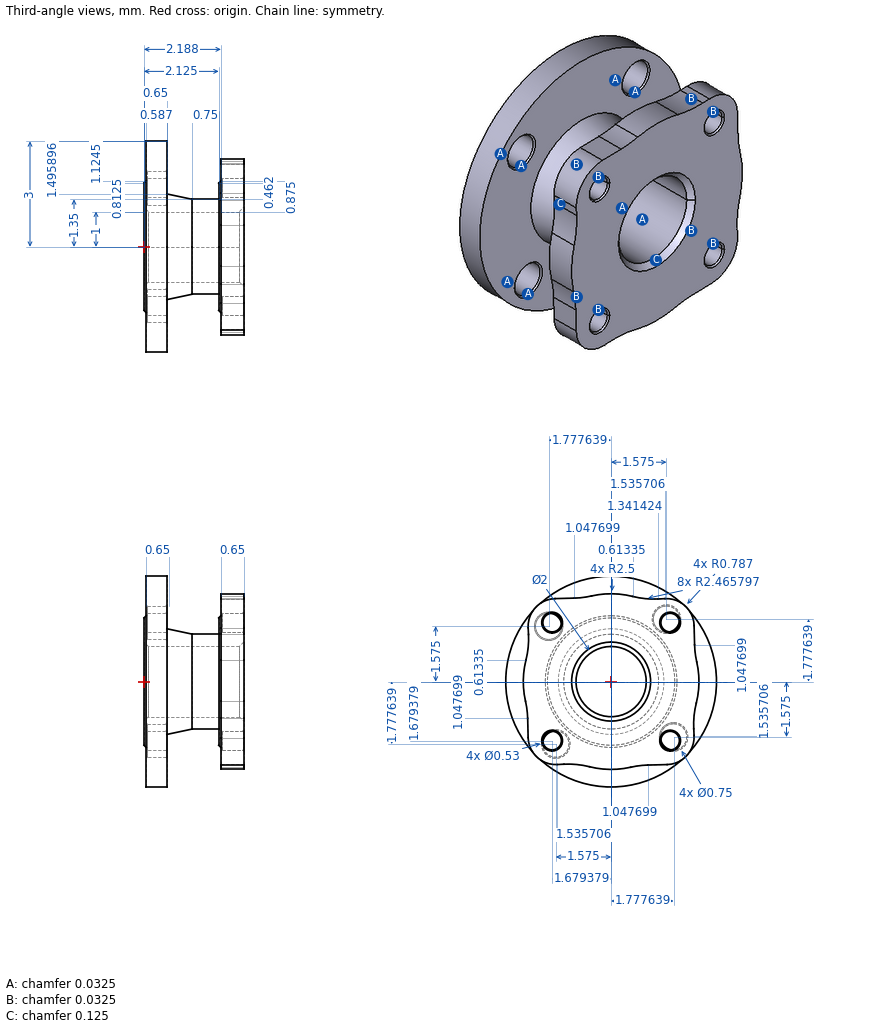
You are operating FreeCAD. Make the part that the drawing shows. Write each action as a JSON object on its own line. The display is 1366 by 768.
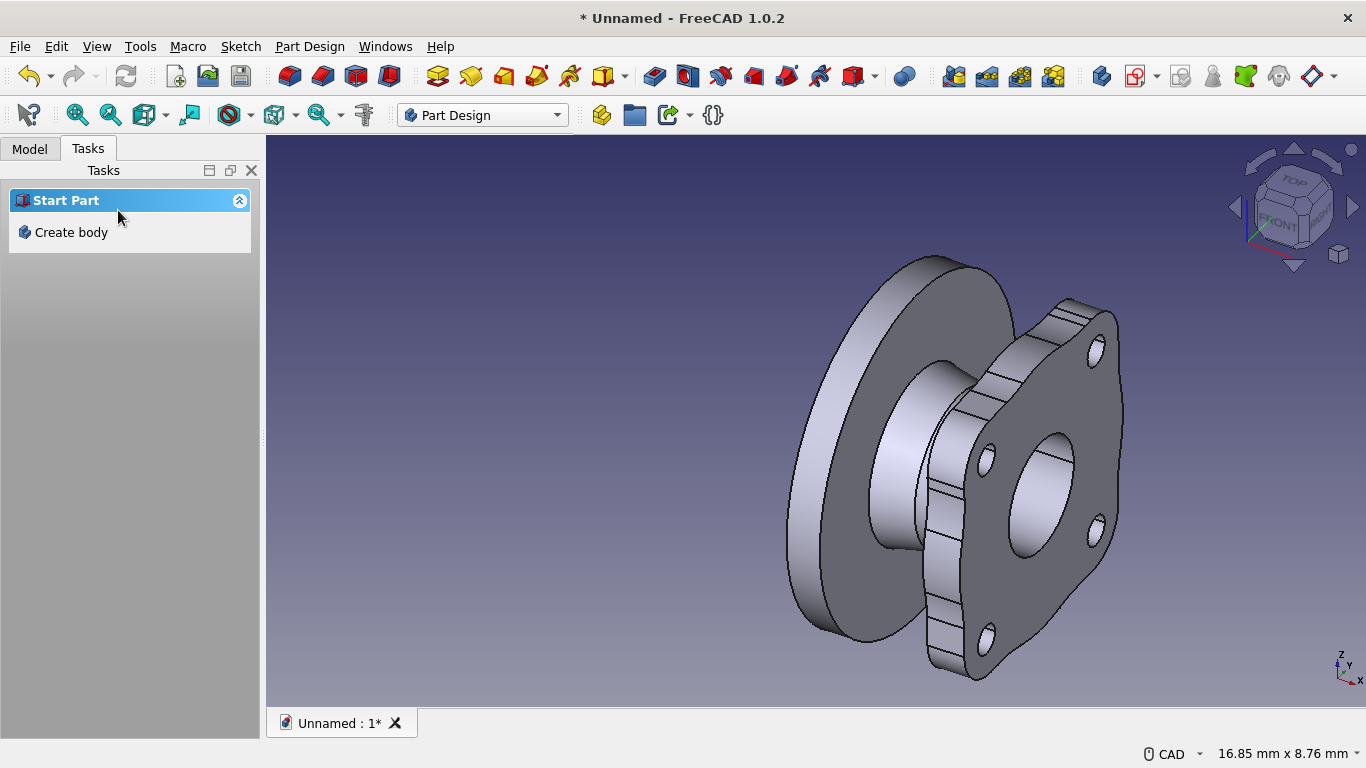
{"action": "left_click", "coordinate": [78, 116]}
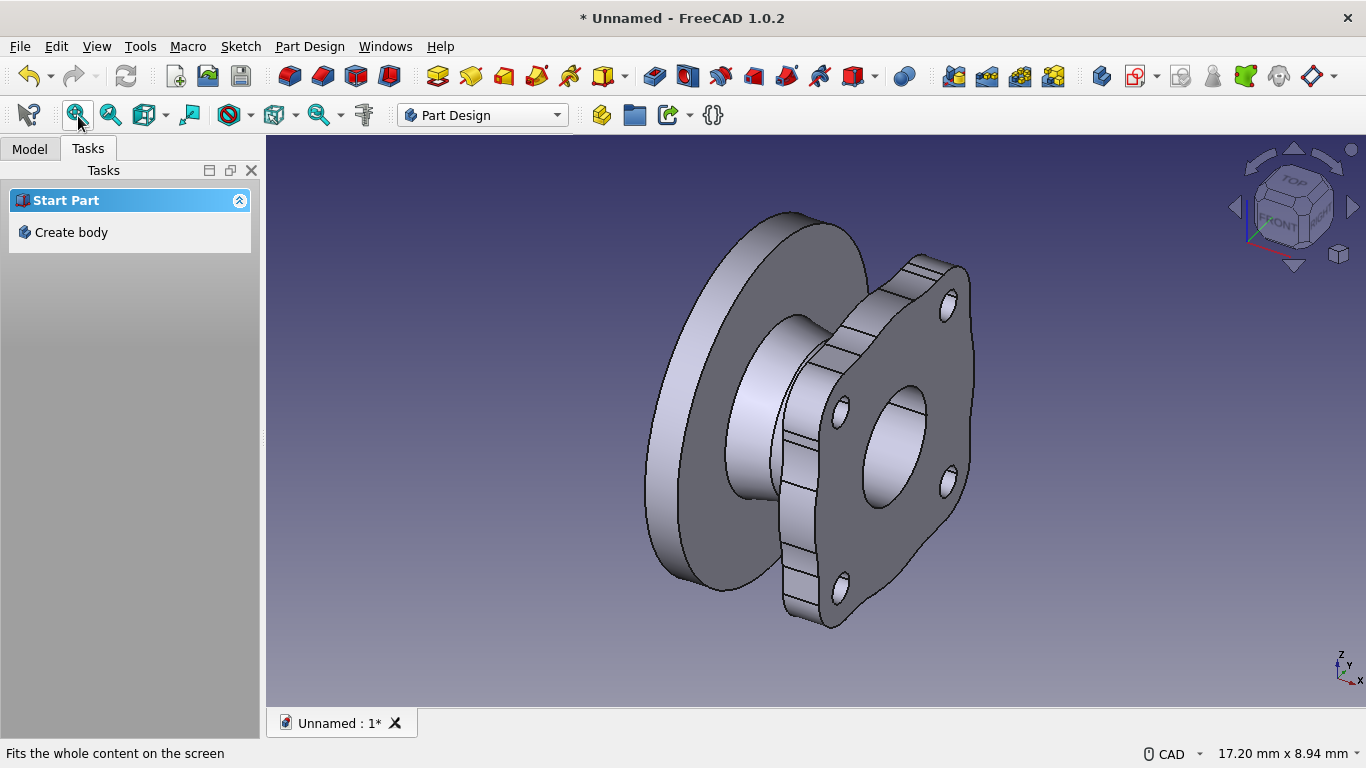
{"action": "key", "text": "6"}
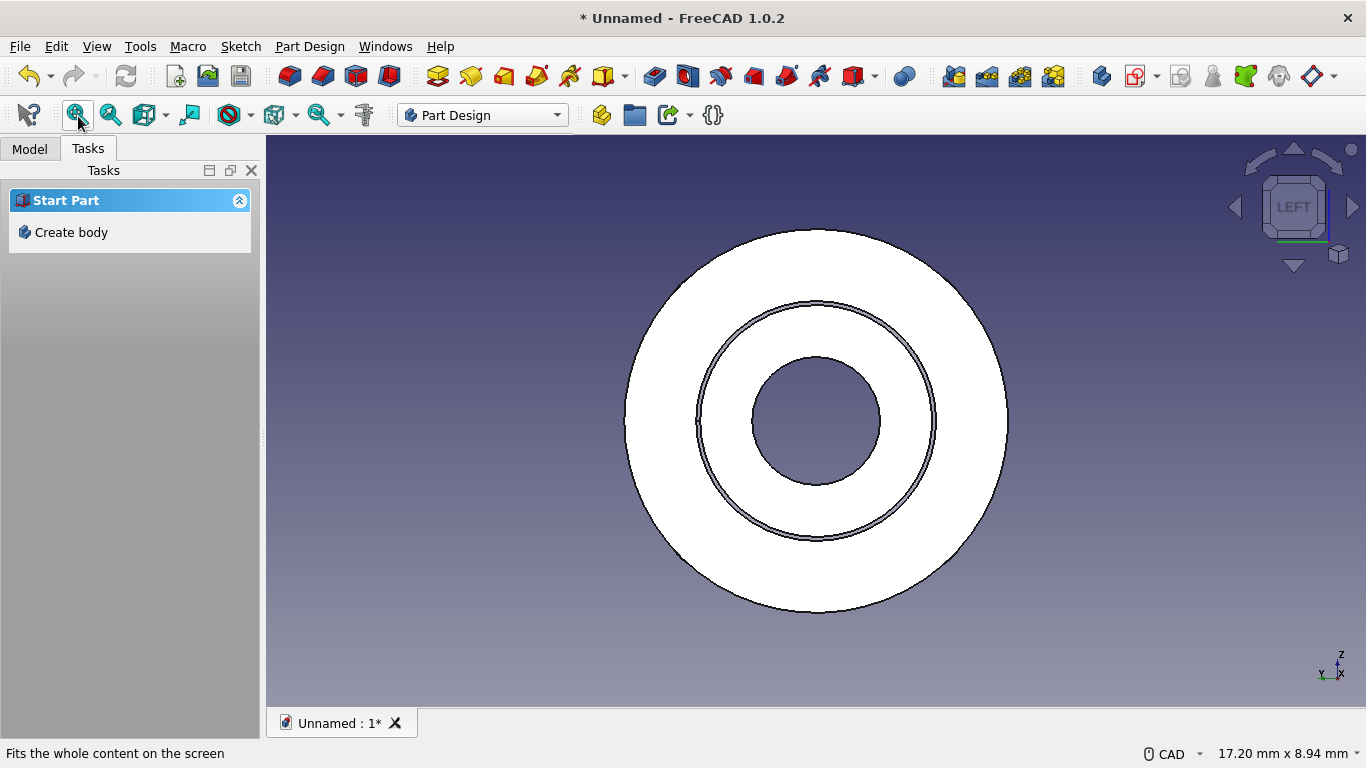
{"action": "left_click", "coordinate": [707, 310]}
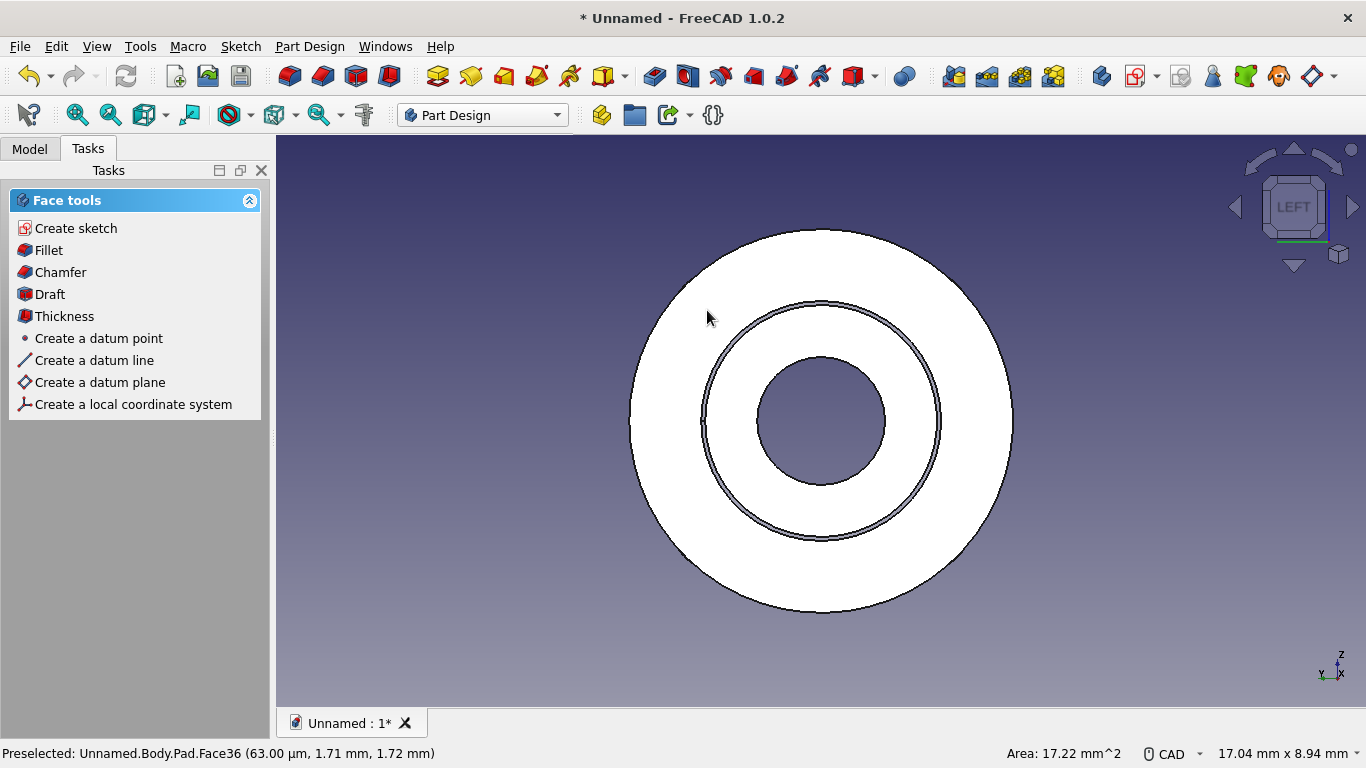
{"action": "left_click", "coordinate": [1134, 76]}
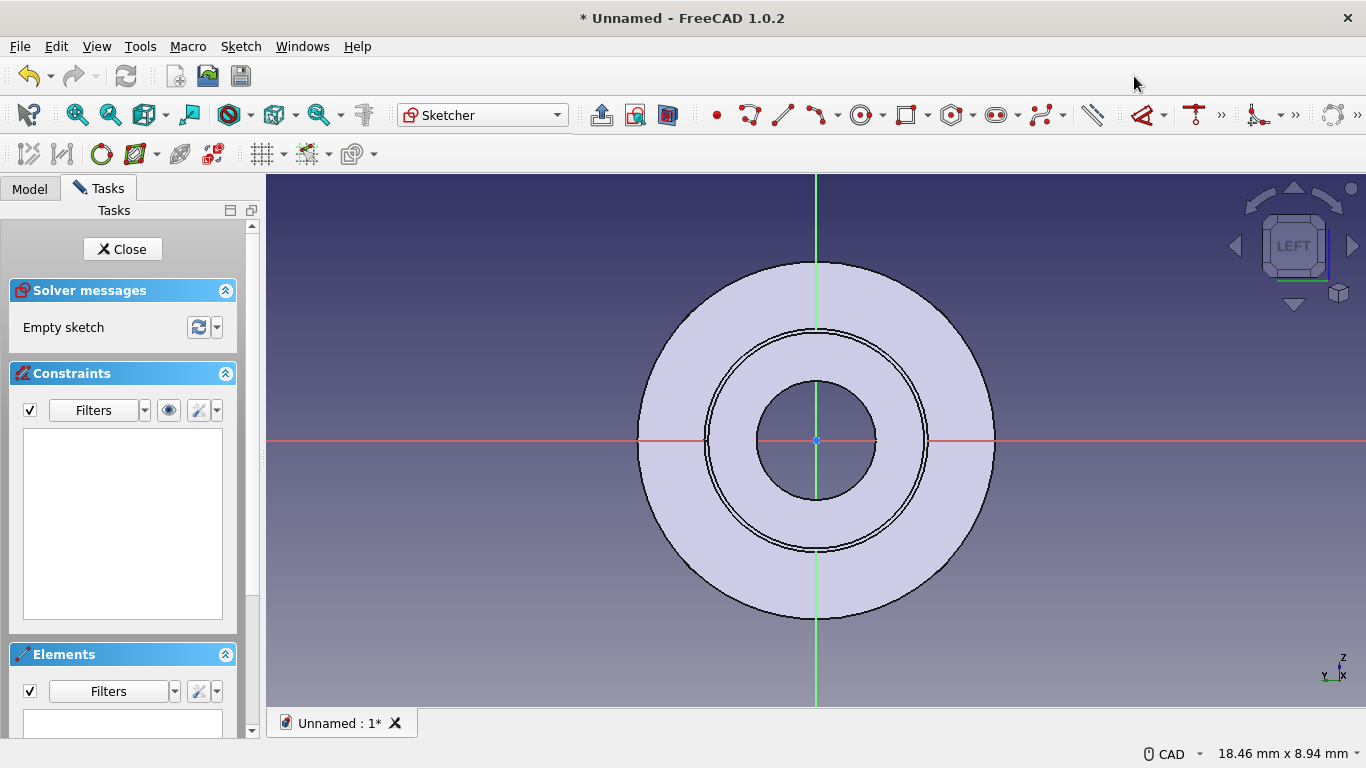
{"action": "left_click", "coordinate": [668, 116]}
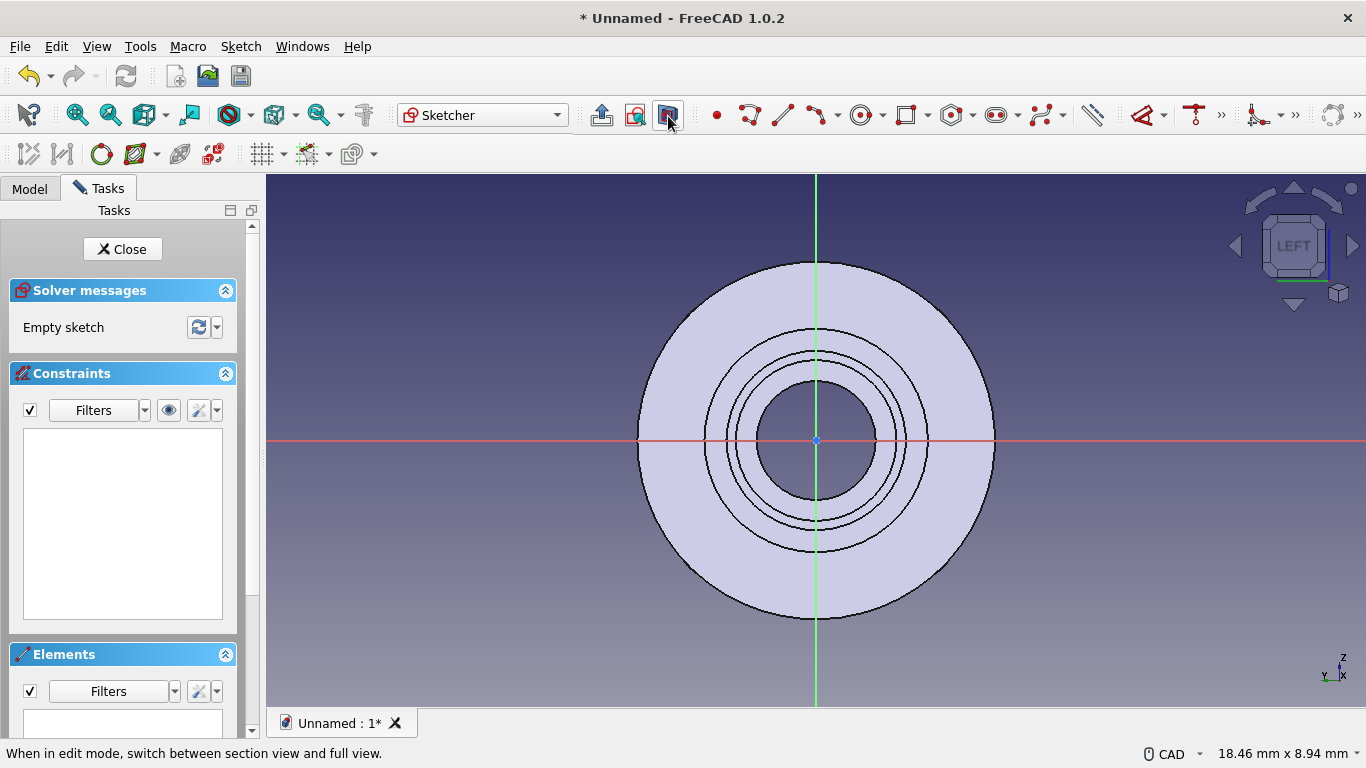
{"action": "left_click", "coordinate": [860, 116]}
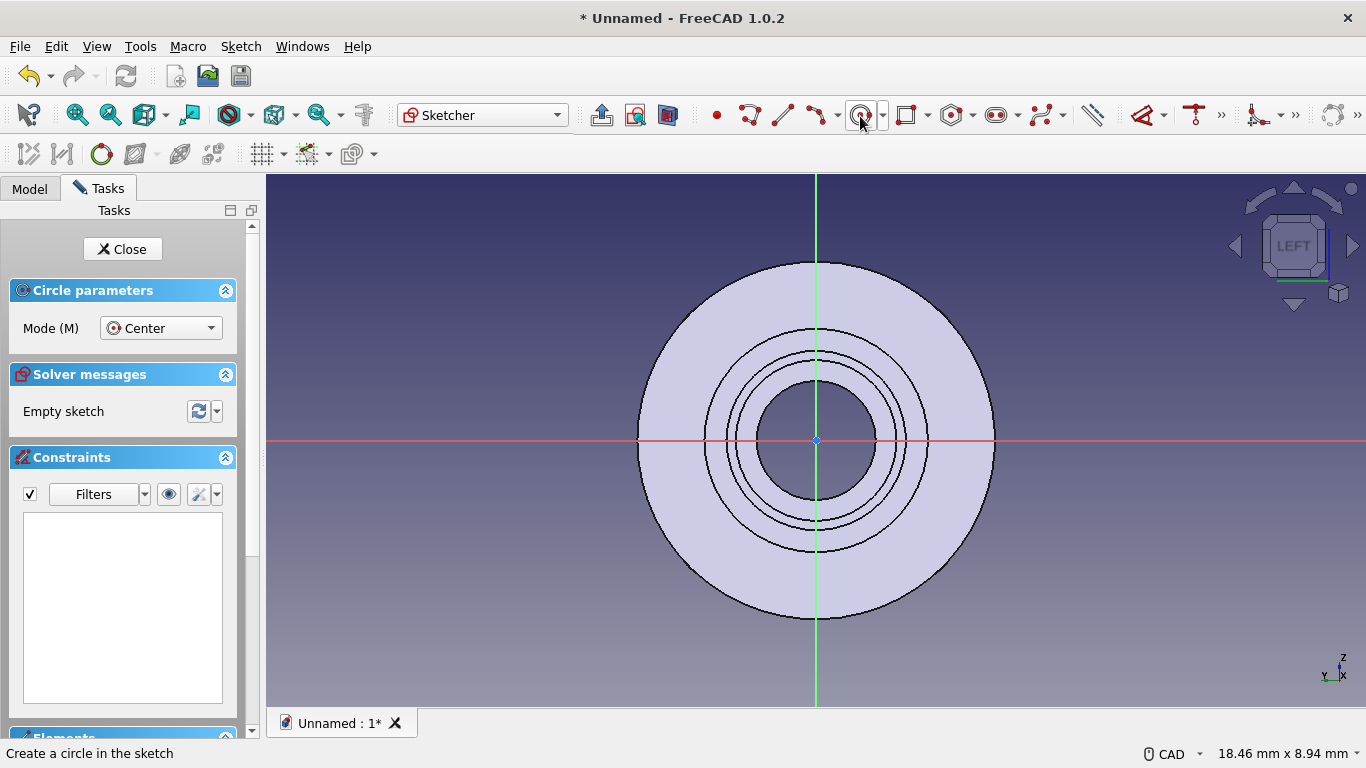
{"action": "left_click", "coordinate": [710, 534]}
{"action": "left_click", "coordinate": [726, 519]}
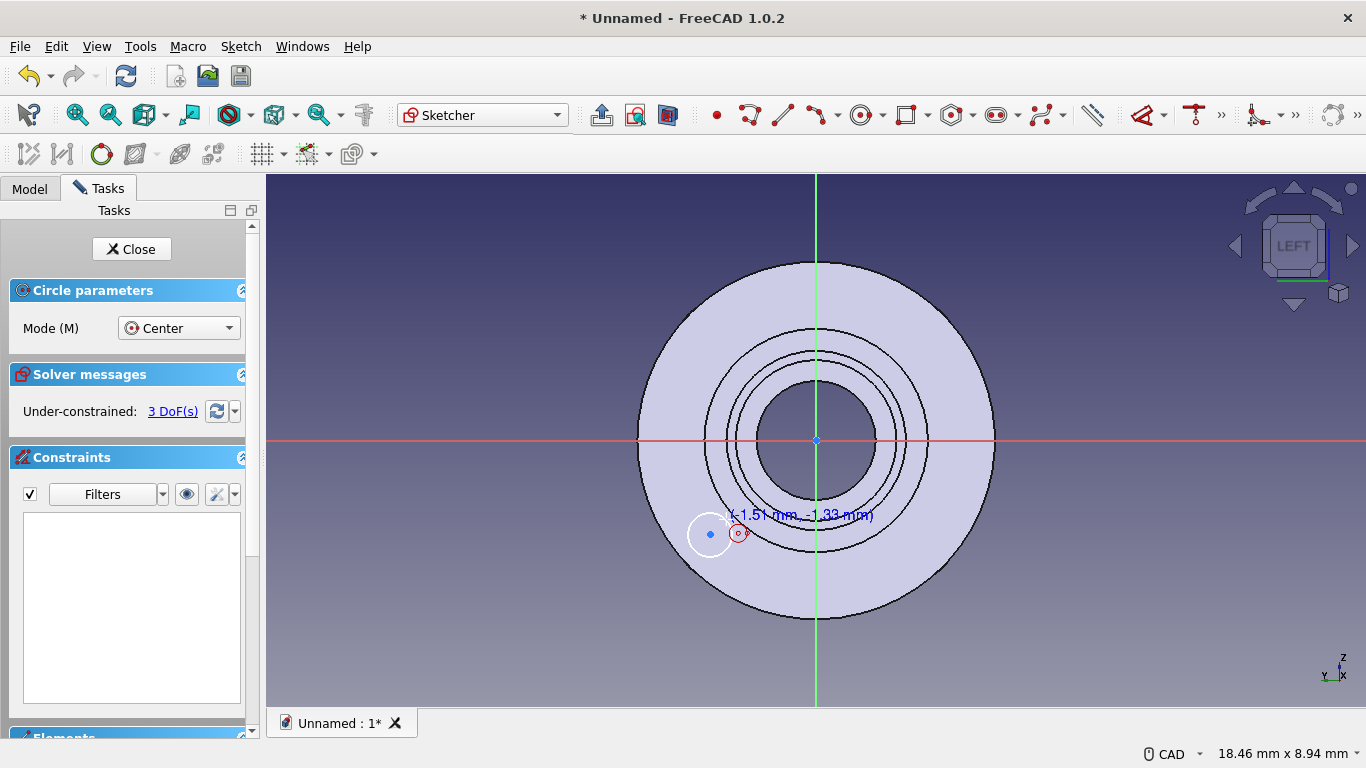
{"action": "left_click", "coordinate": [722, 335]}
{"action": "left_click", "coordinate": [738, 319]}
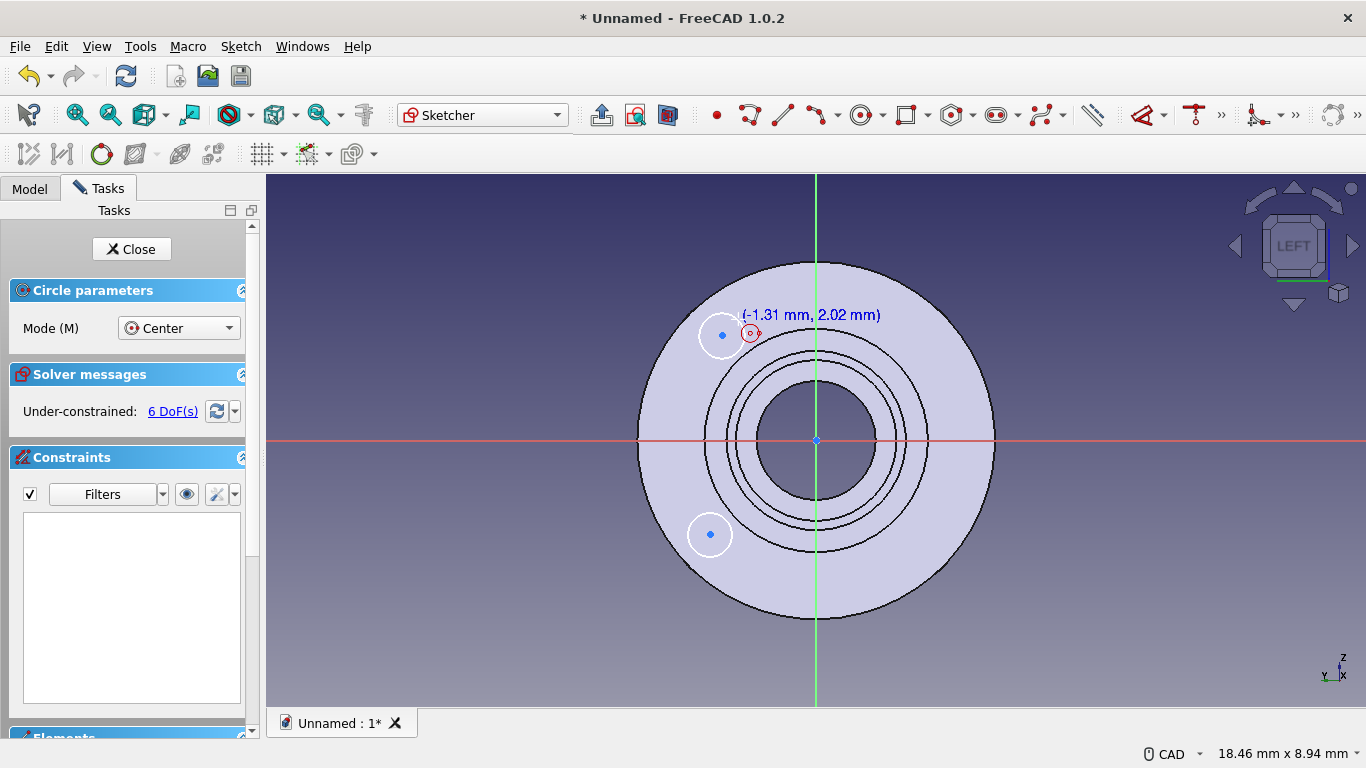
{"action": "left_click", "coordinate": [922, 347]}
{"action": "left_click", "coordinate": [938, 331]}